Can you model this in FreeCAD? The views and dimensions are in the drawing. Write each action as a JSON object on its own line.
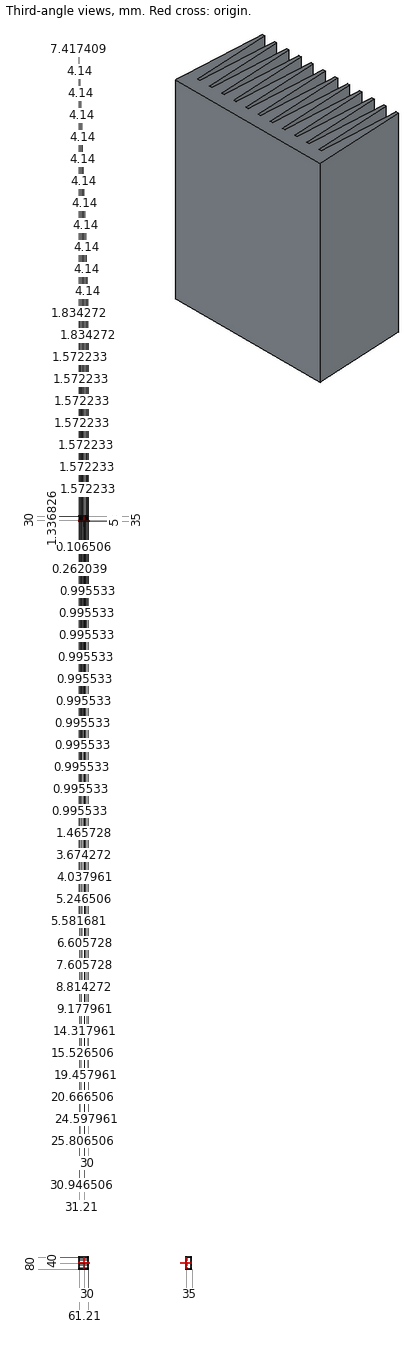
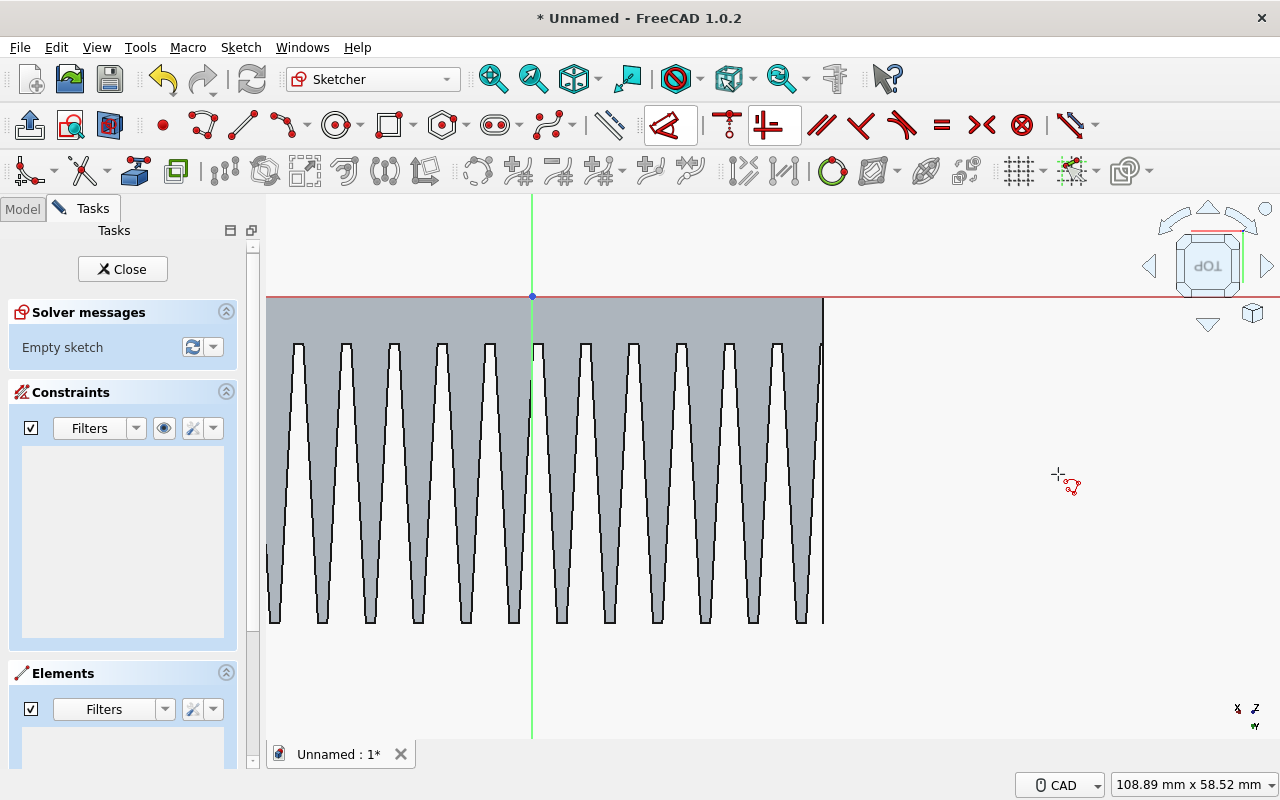
{"action": "left_click", "coordinate": [823, 297]}
{"action": "left_click", "coordinate": [806, 623]}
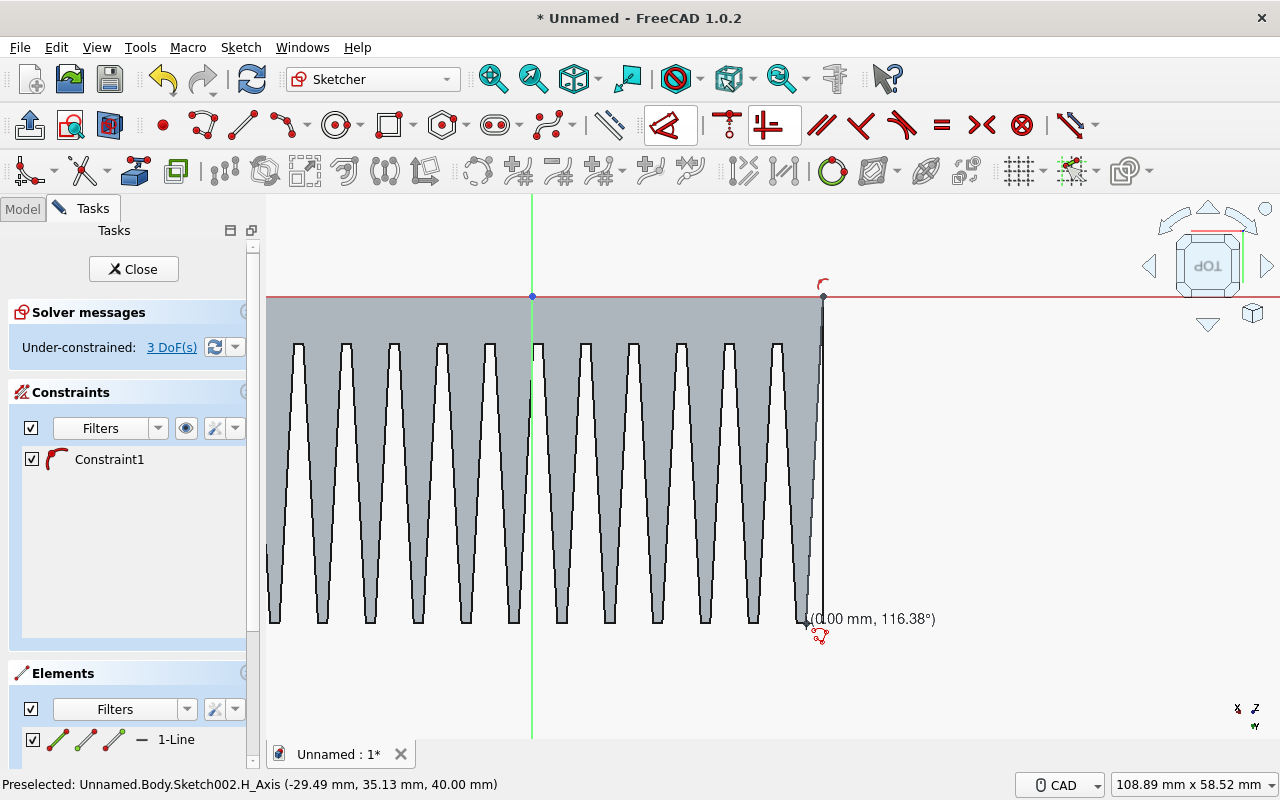
{"action": "scroll", "coordinate": [806, 635], "scroll_direction": "up", "scroll_amount": 2}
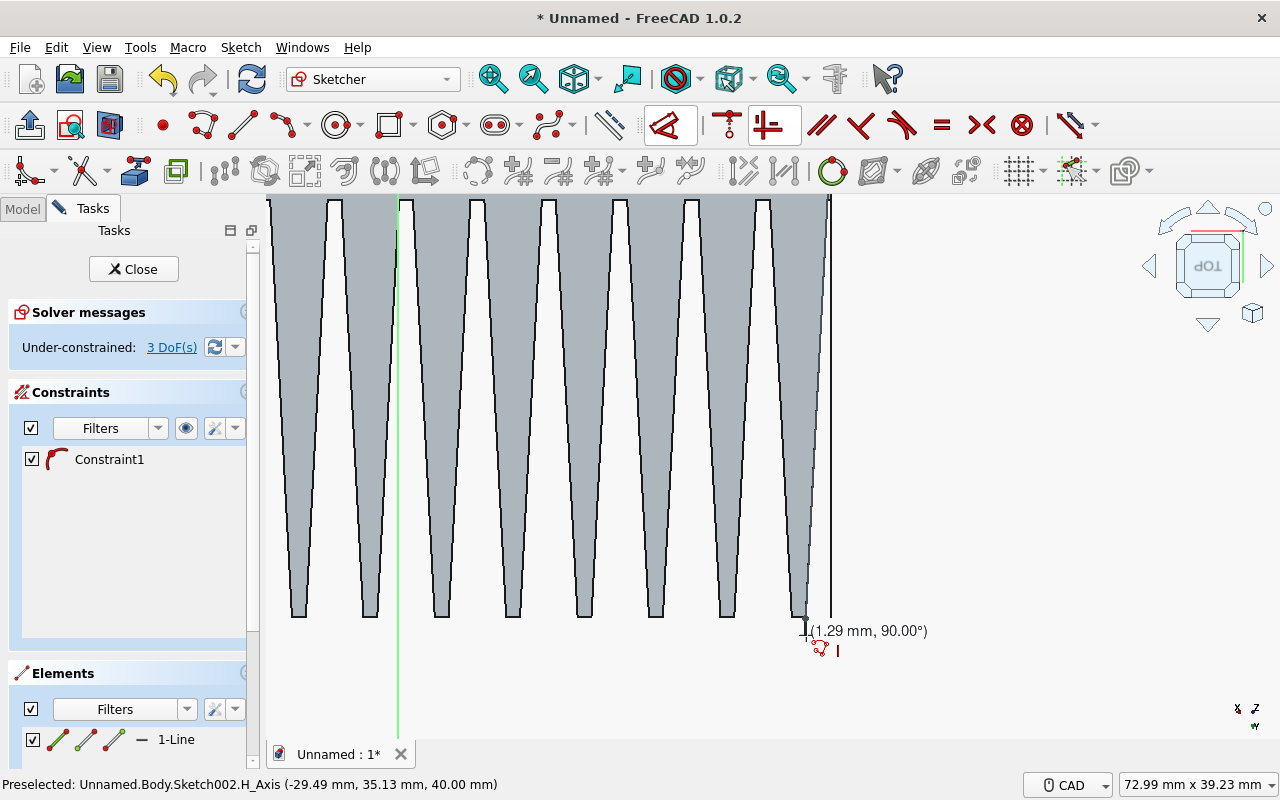
{"action": "left_click", "coordinate": [806, 635]}
{"action": "left_click", "coordinate": [909, 635]}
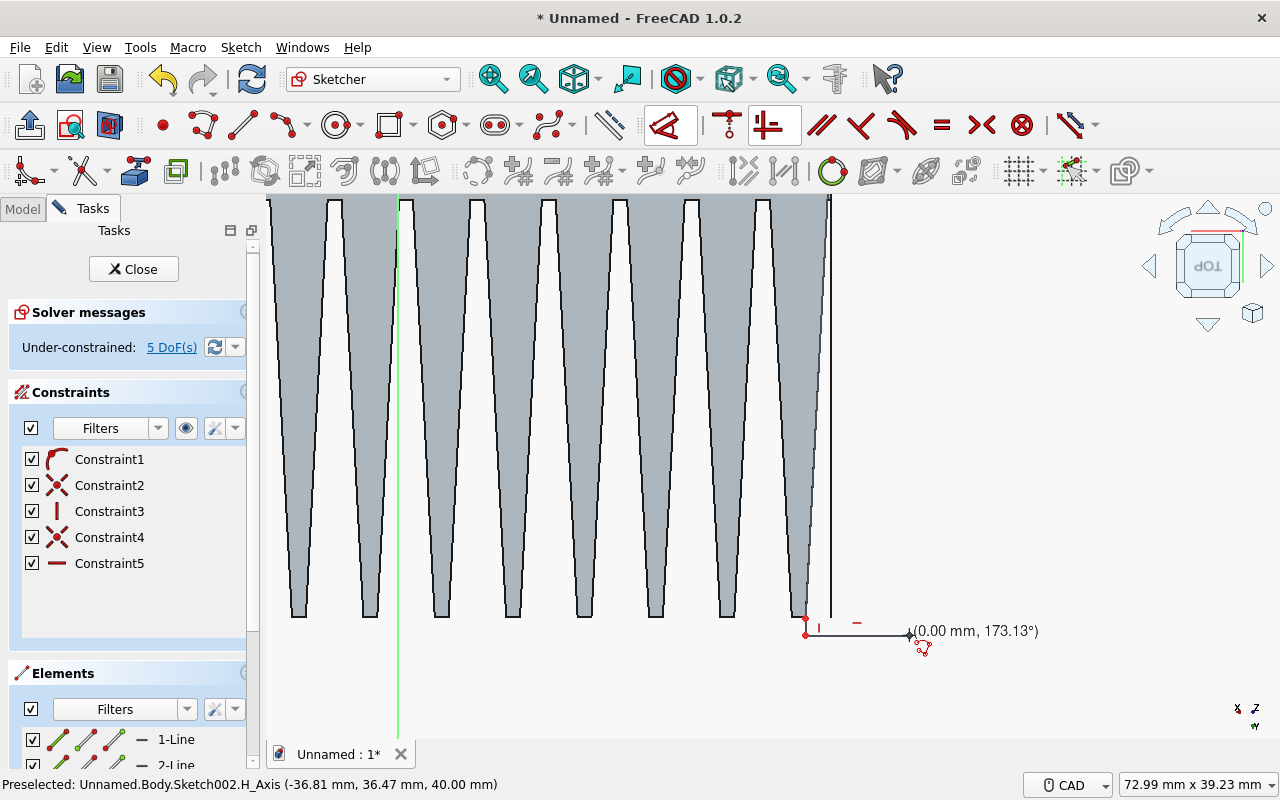
{"action": "scroll", "coordinate": [809, 637], "scroll_direction": "down", "scroll_amount": 2}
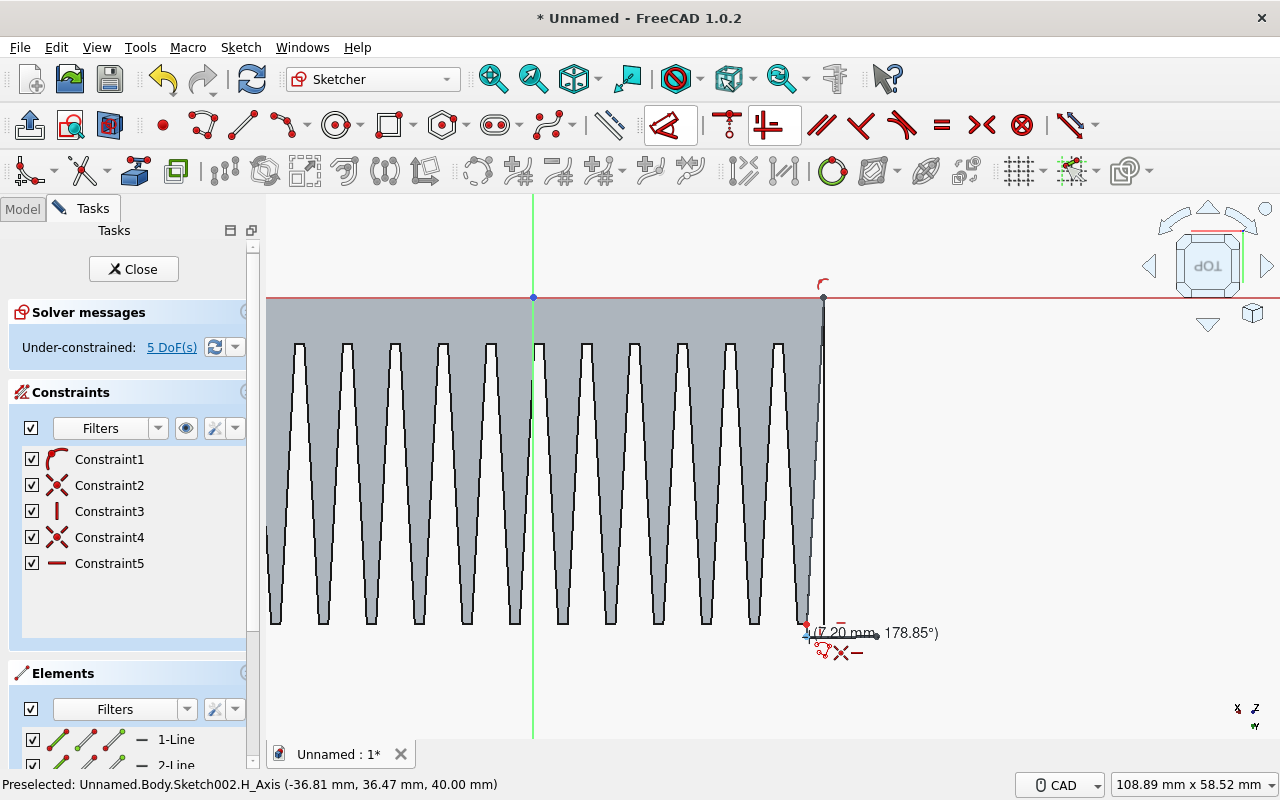
{"action": "left_click", "coordinate": [876, 307]}
{"action": "left_click", "coordinate": [824, 298]}
{"action": "key", "text": "Escape"}
{"action": "key", "text": "Escape"}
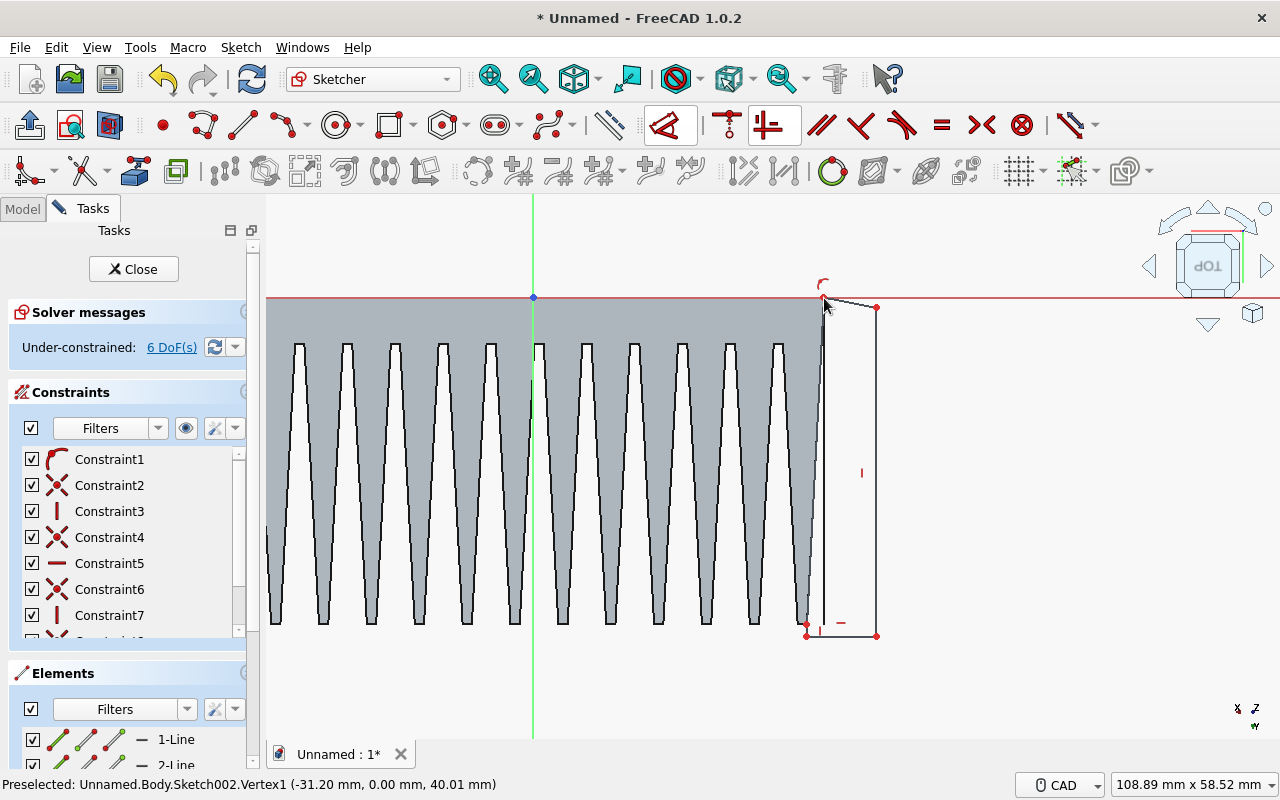
{"action": "left_click", "coordinate": [840, 301]}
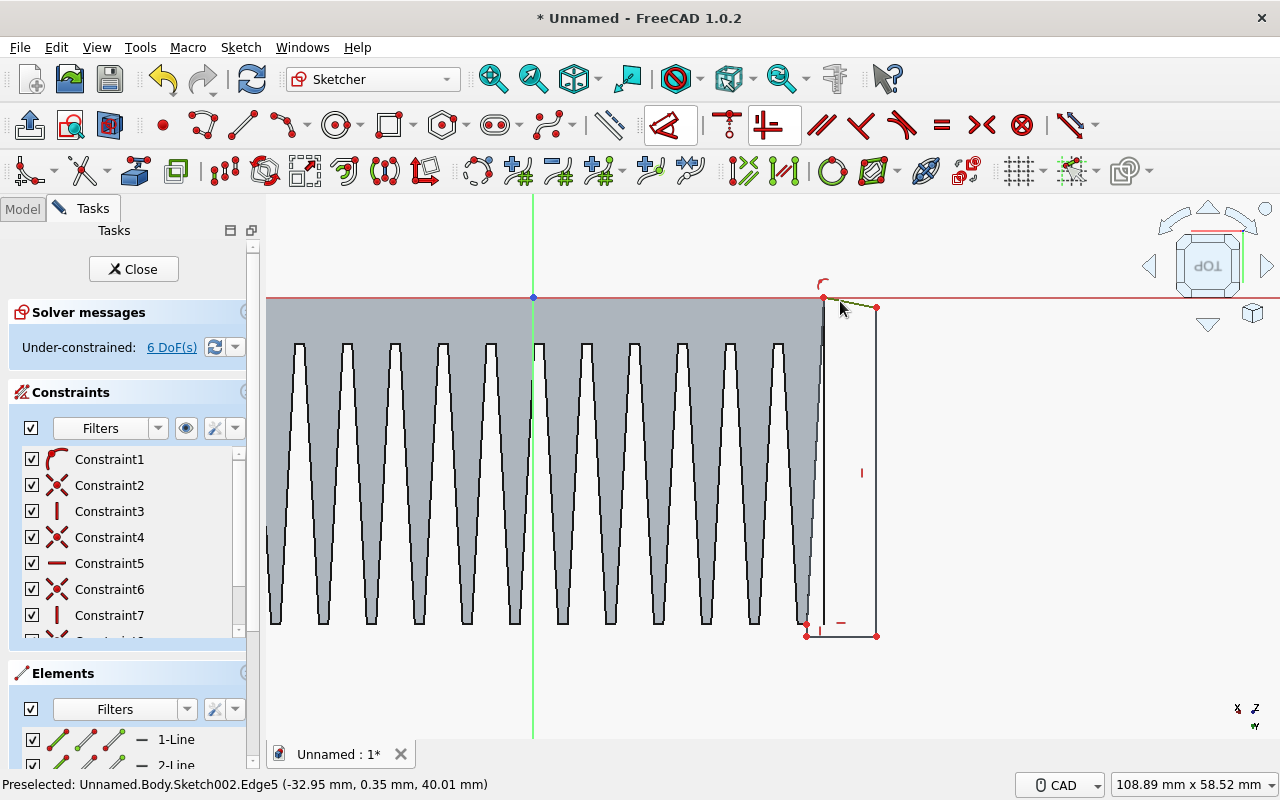
{"action": "key", "text": "h"}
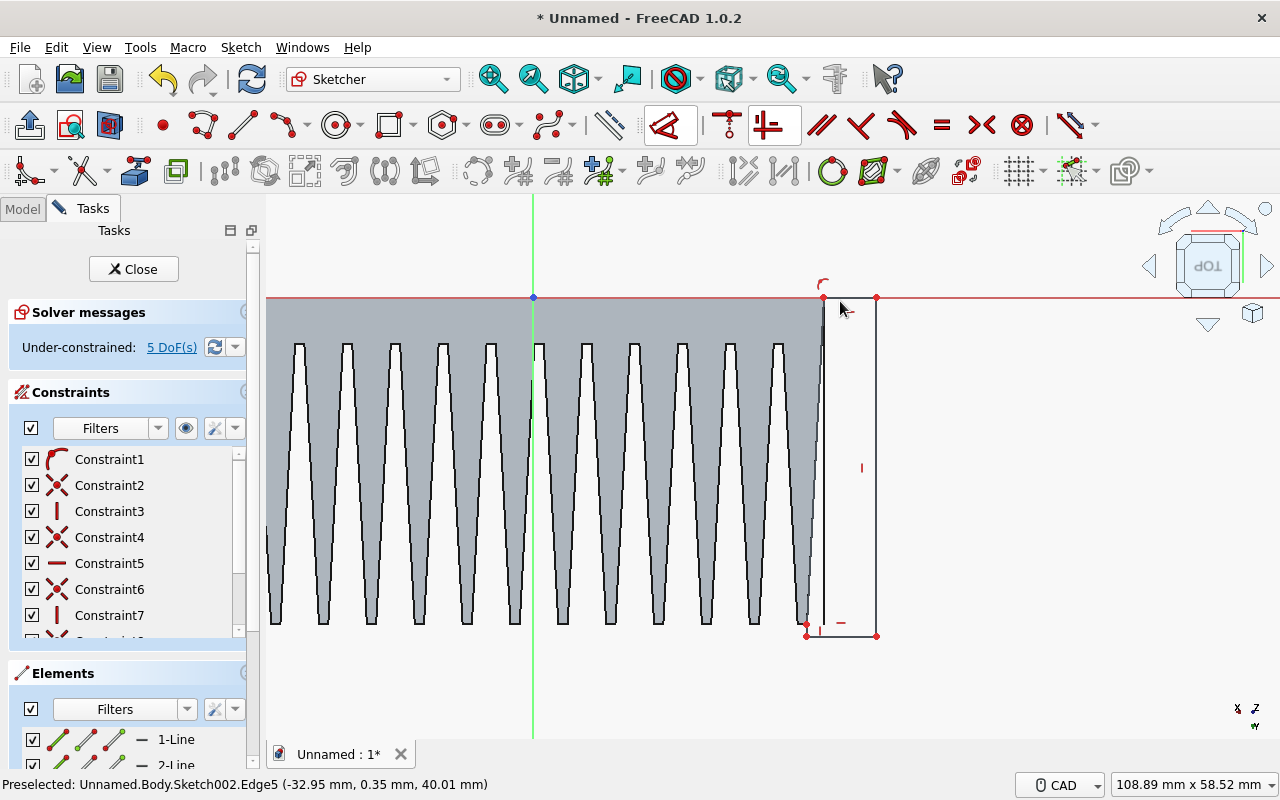
{"action": "left_click", "coordinate": [807, 625]}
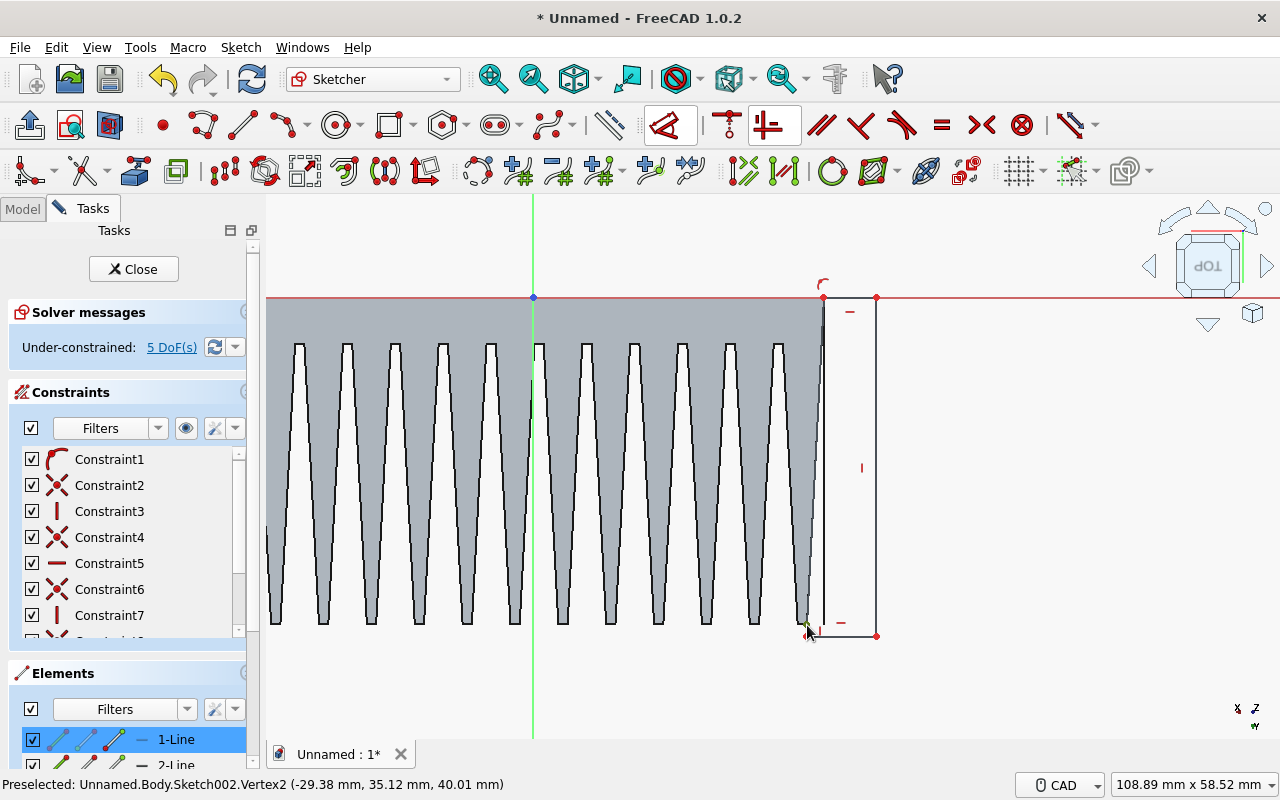
{"action": "key", "text": "i"}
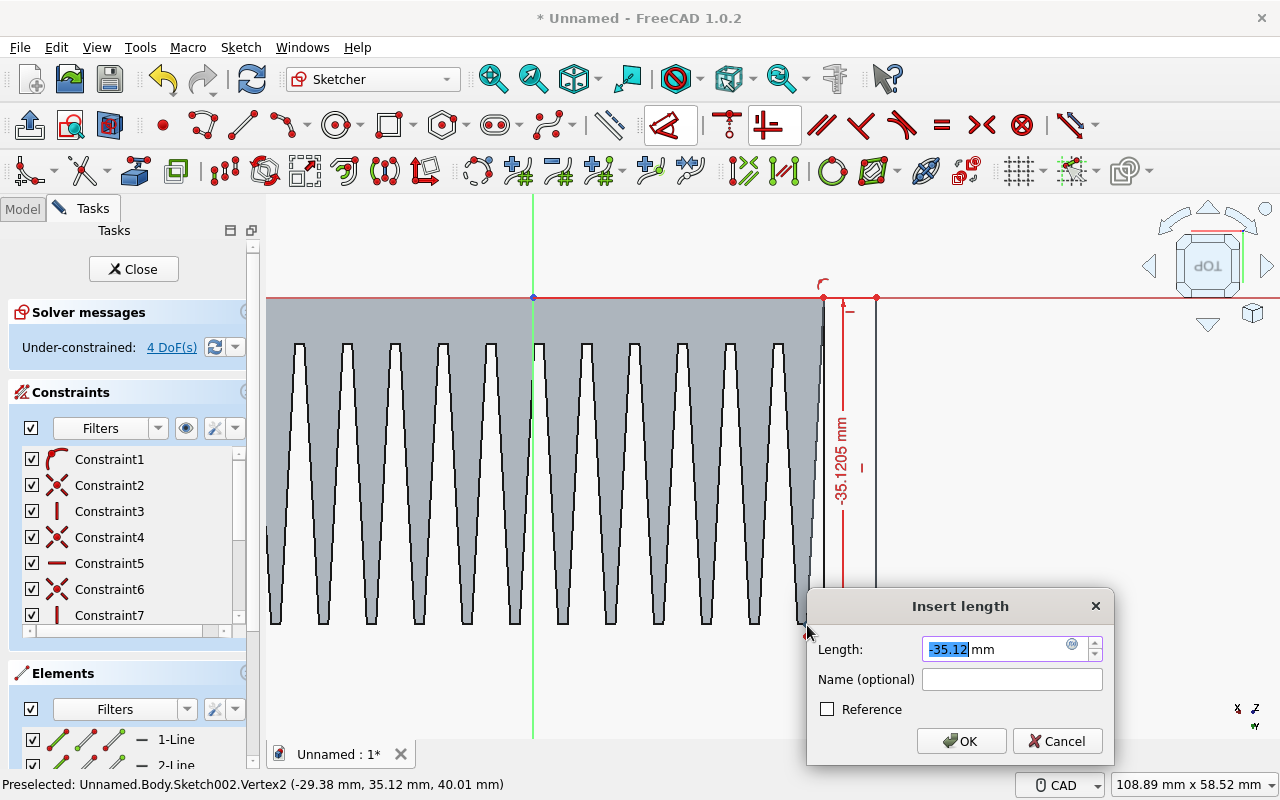
{"action": "type", "text": "-35"}
{"action": "key", "text": "Return"}